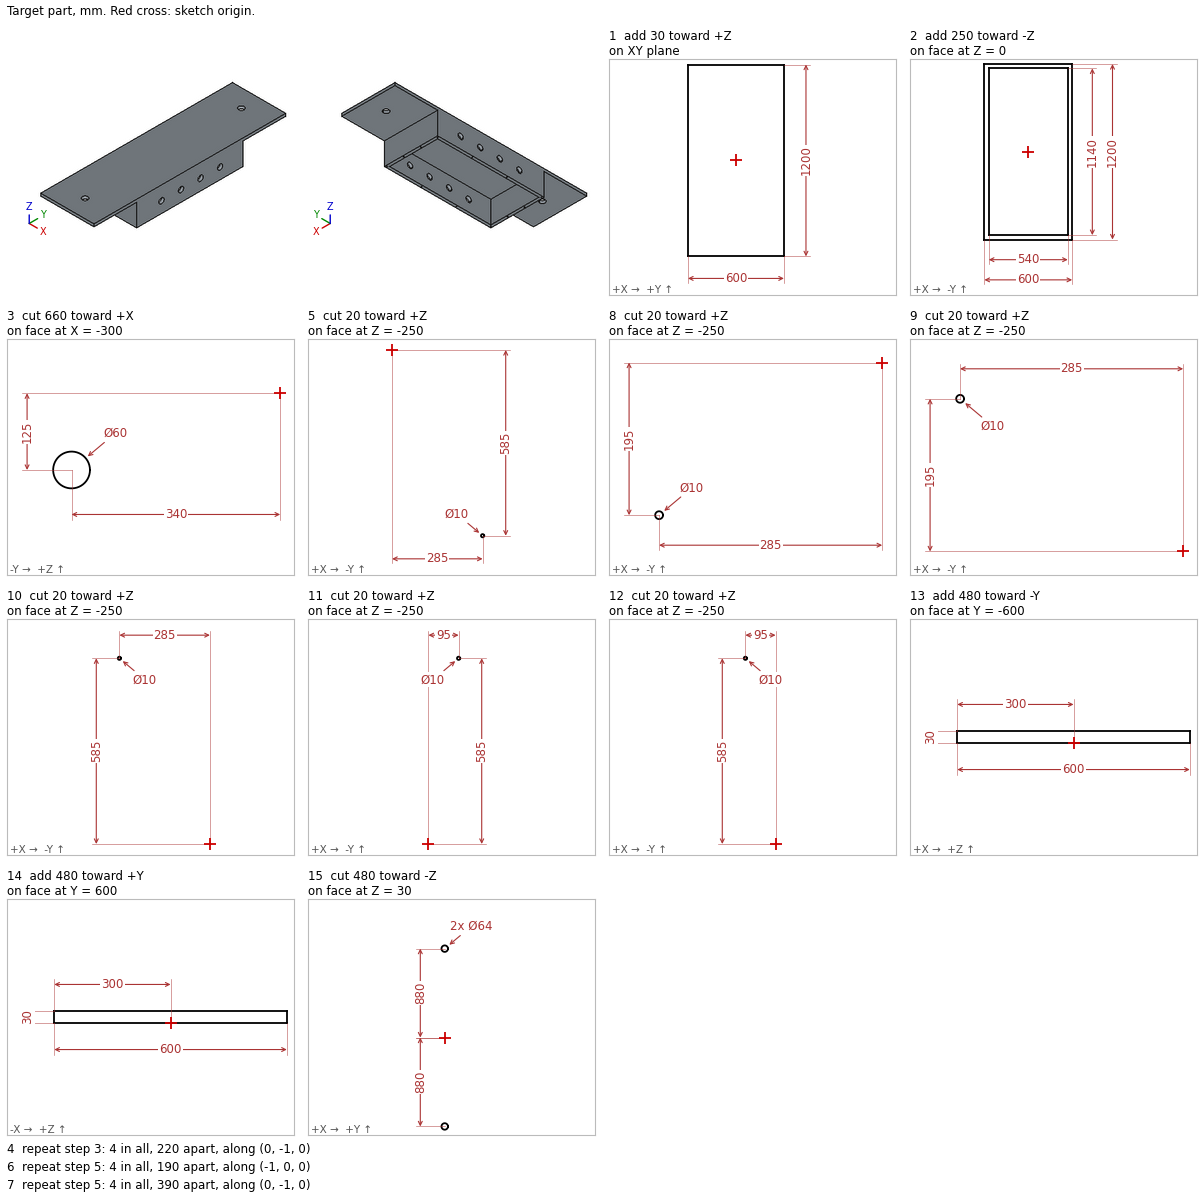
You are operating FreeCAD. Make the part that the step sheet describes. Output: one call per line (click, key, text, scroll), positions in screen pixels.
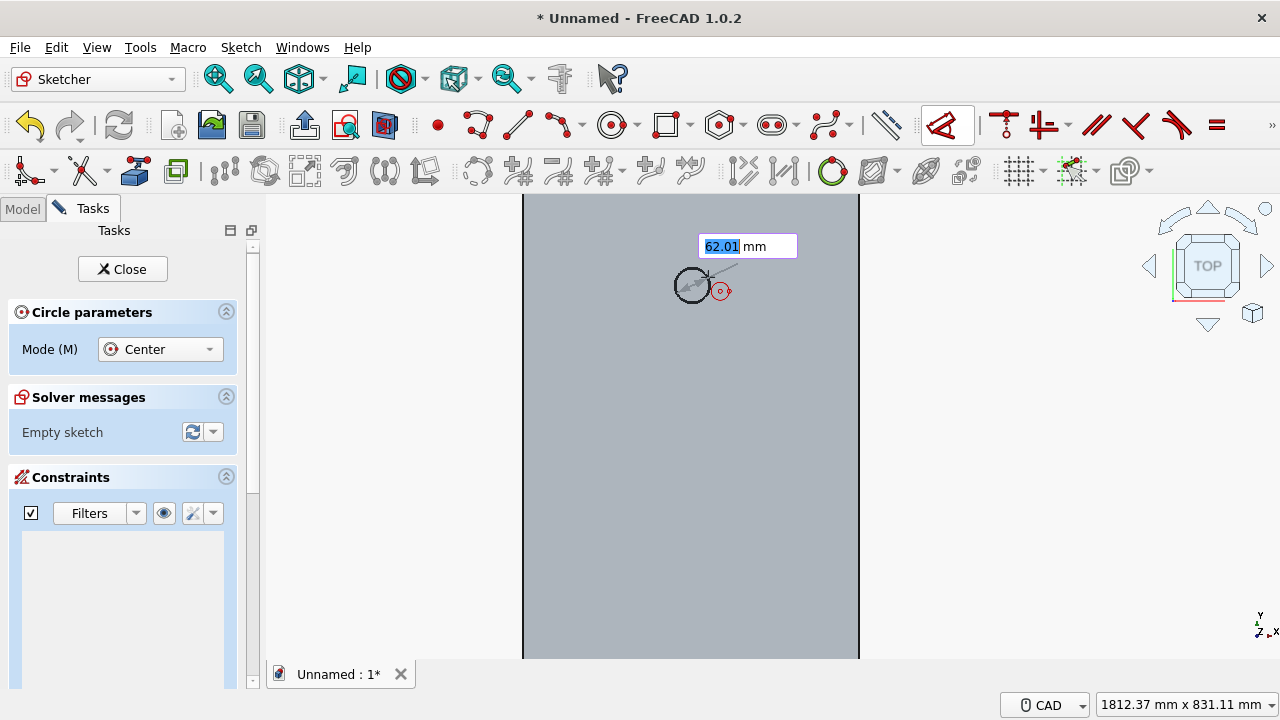
text(64)
key(Return)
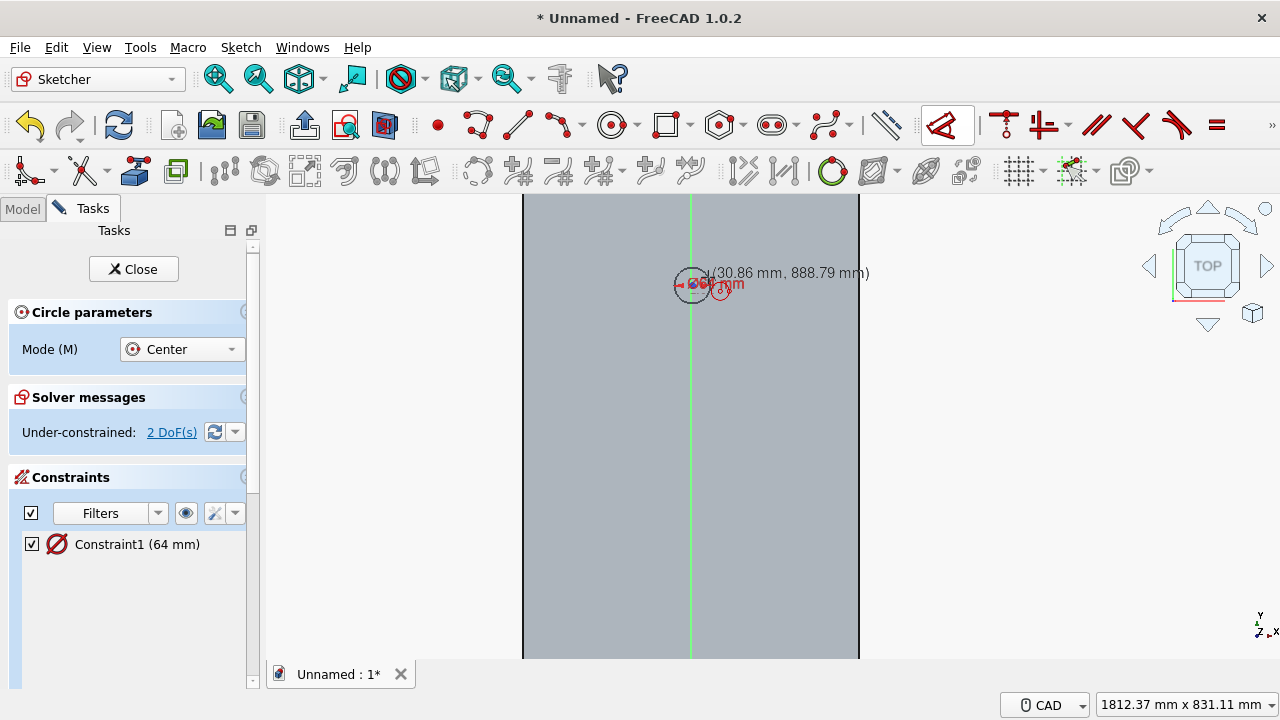
scroll(710, 276, down, 6)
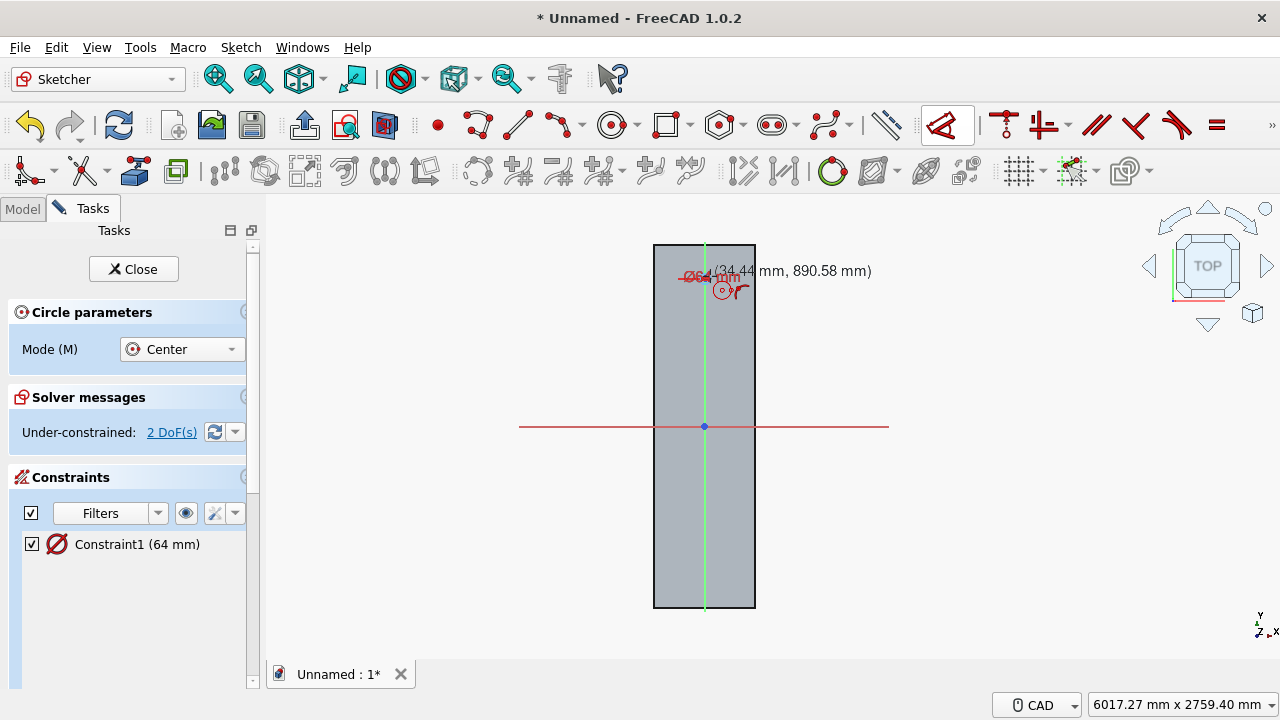
scroll(705, 575, up, 8)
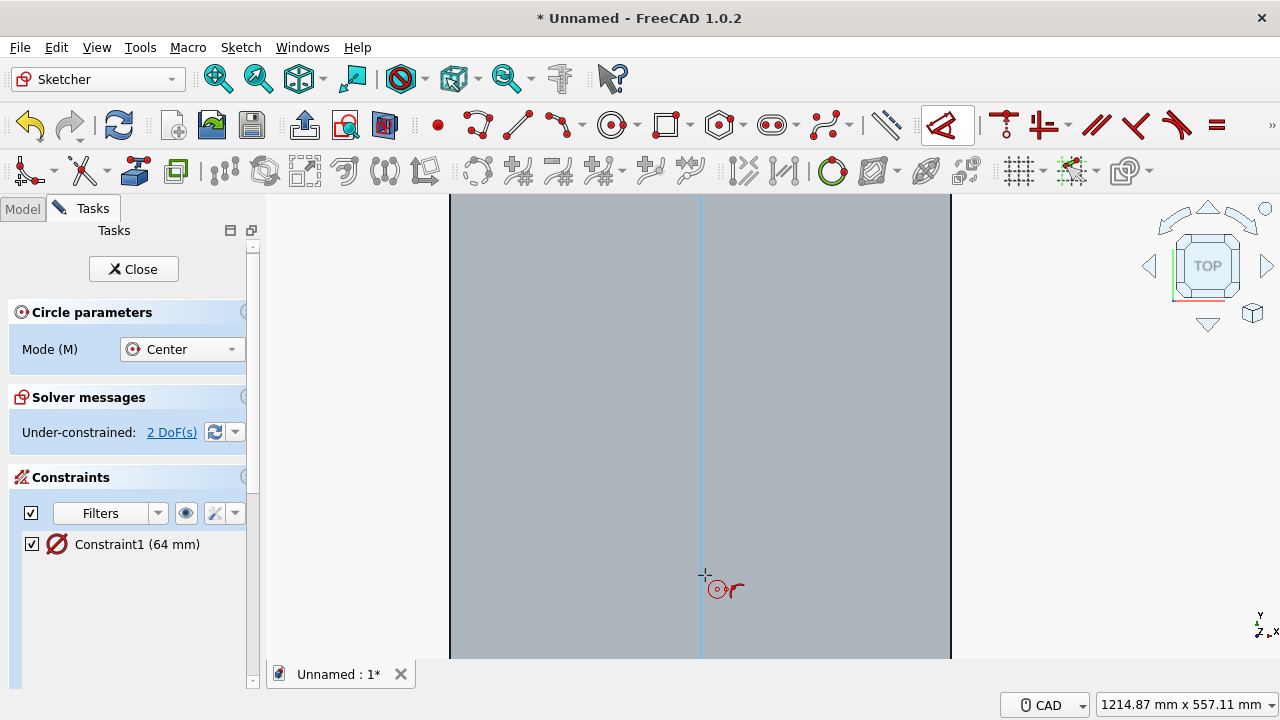
scroll(705, 576, down, 8)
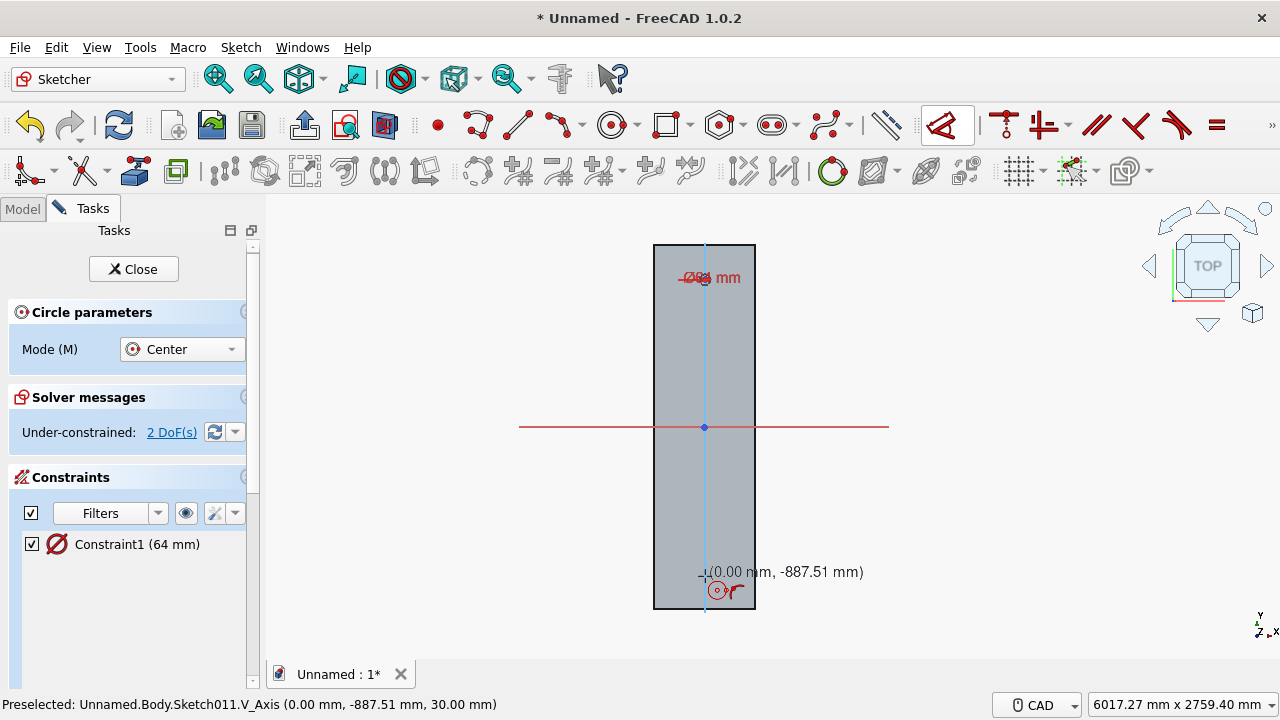
click(705, 576)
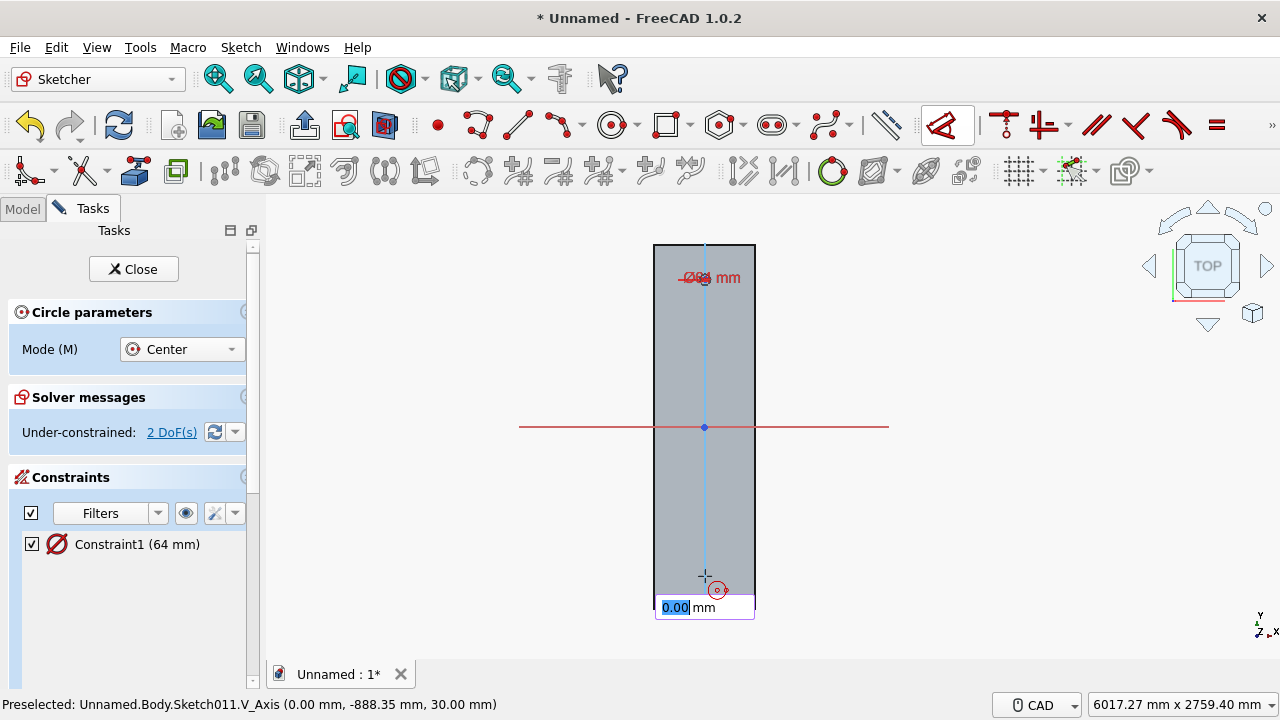
scroll(710, 574, up, 6)
move(708, 571)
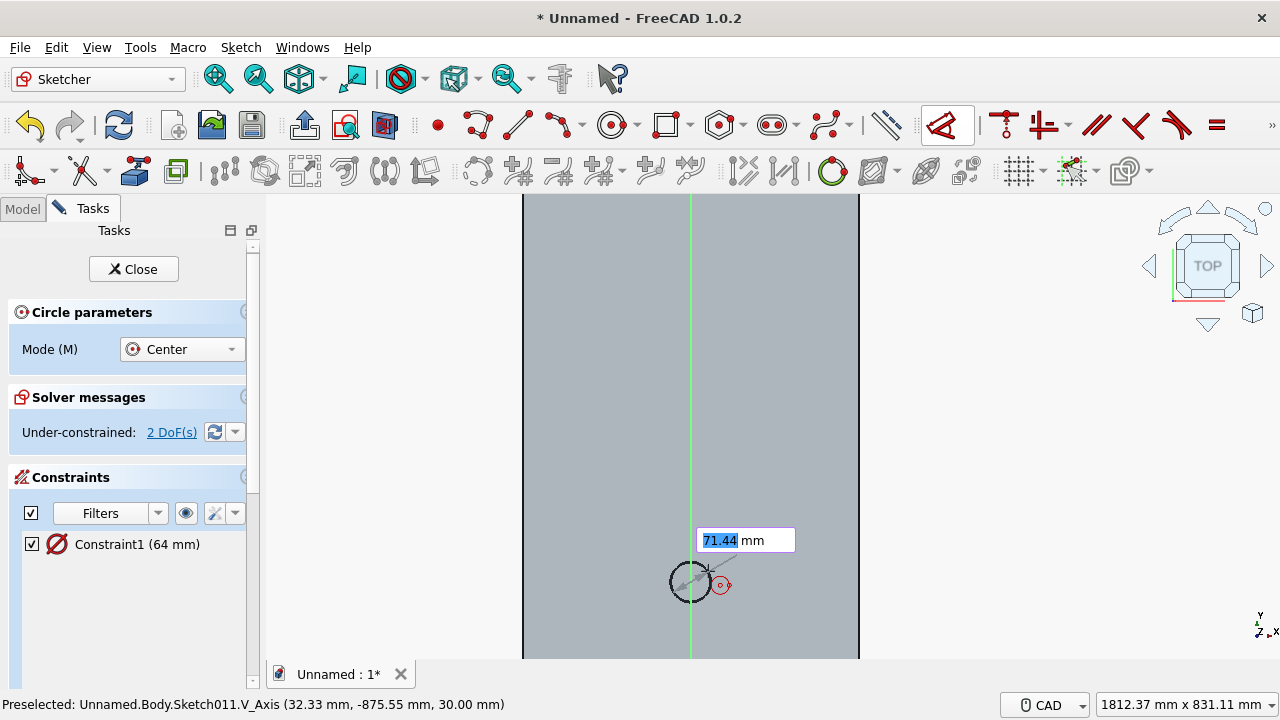
text(64)
key(Return)
key(Escape)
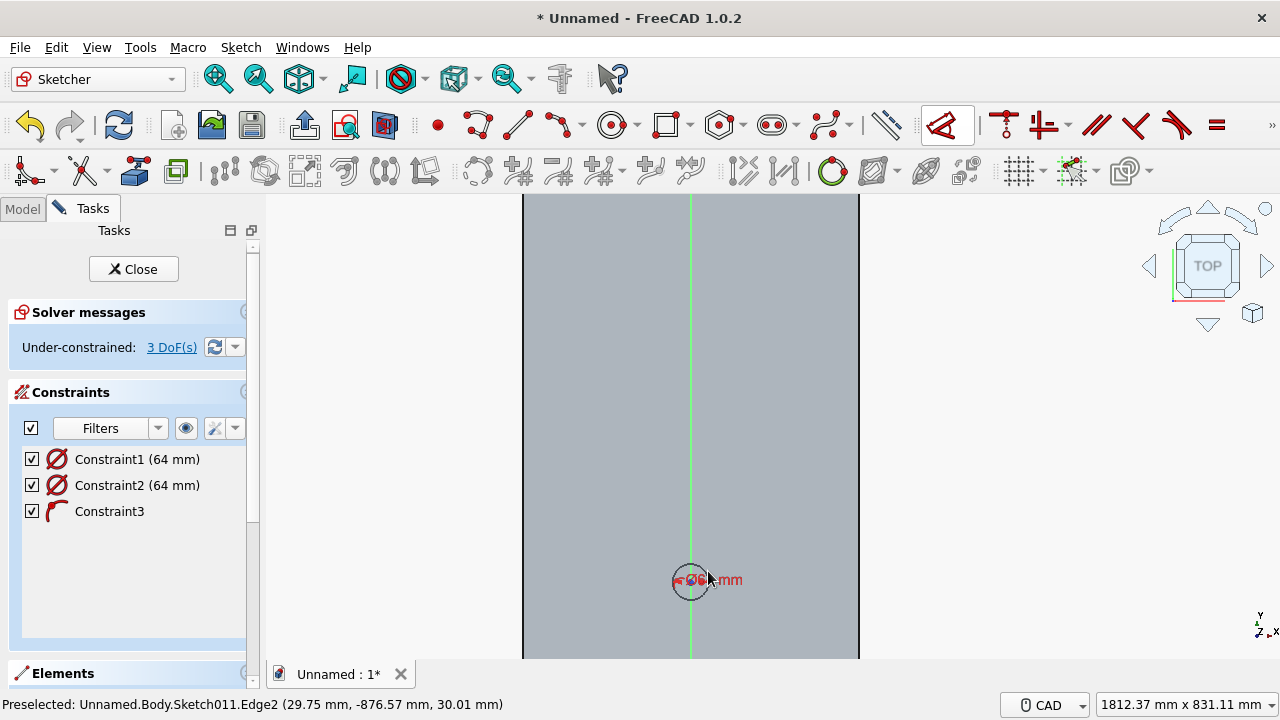
scroll(710, 574, down, 6)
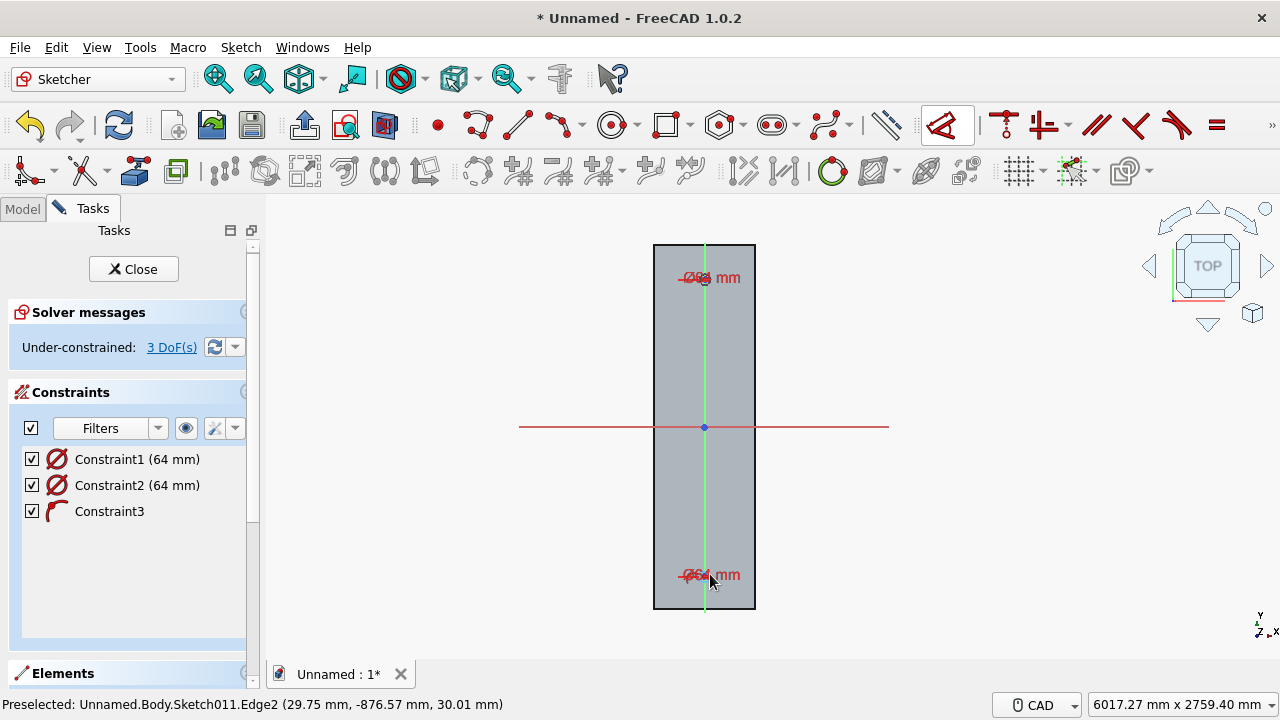
click(705, 280)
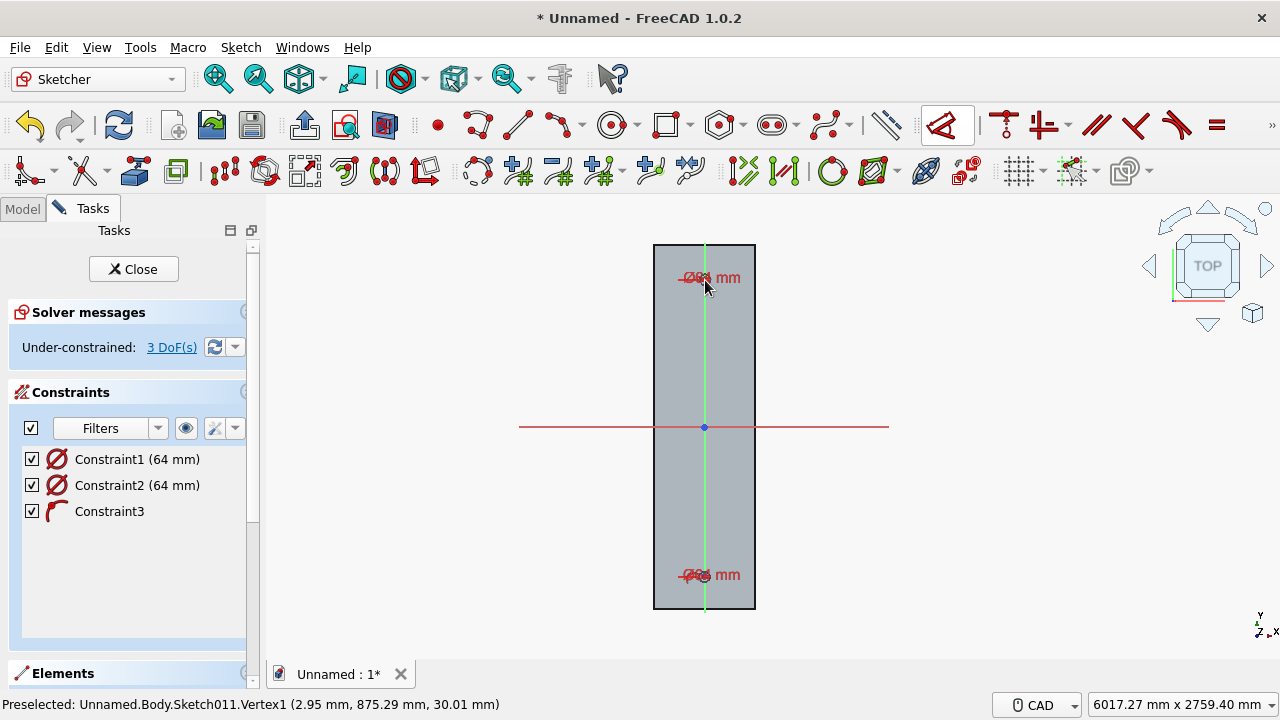
click(705, 514)